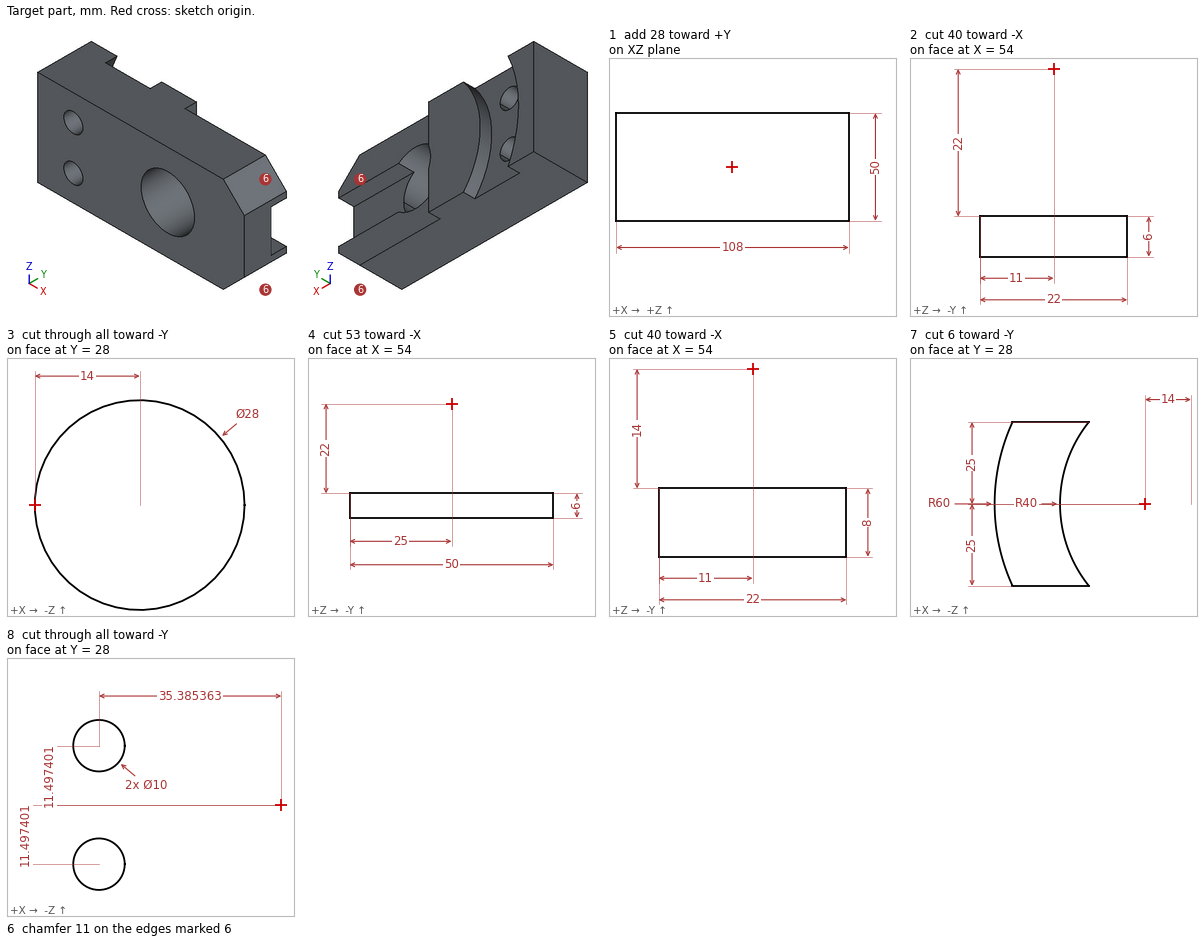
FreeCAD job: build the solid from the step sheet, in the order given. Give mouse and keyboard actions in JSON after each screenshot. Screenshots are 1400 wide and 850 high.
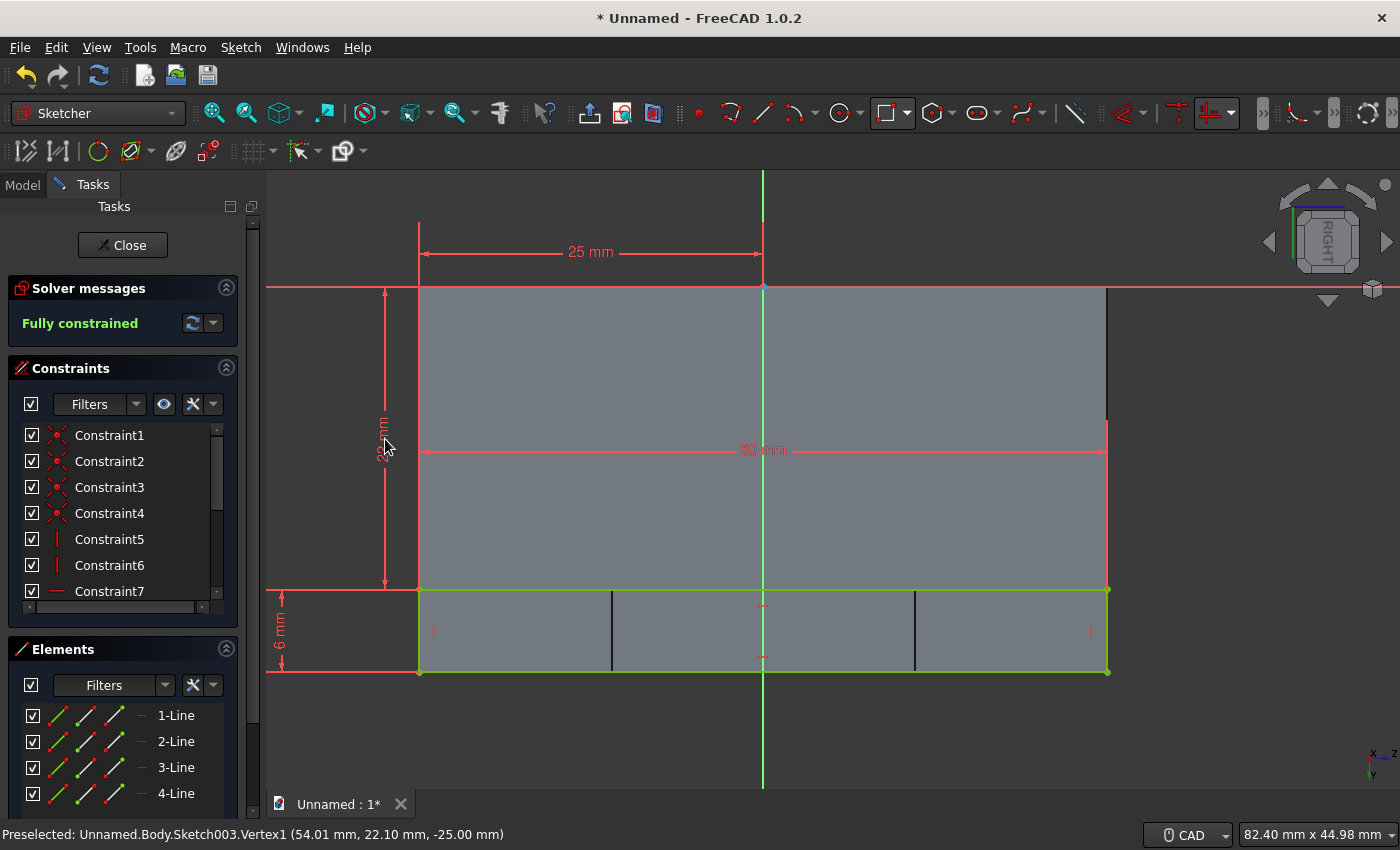
{"action": "left_click", "coordinate": [123, 245]}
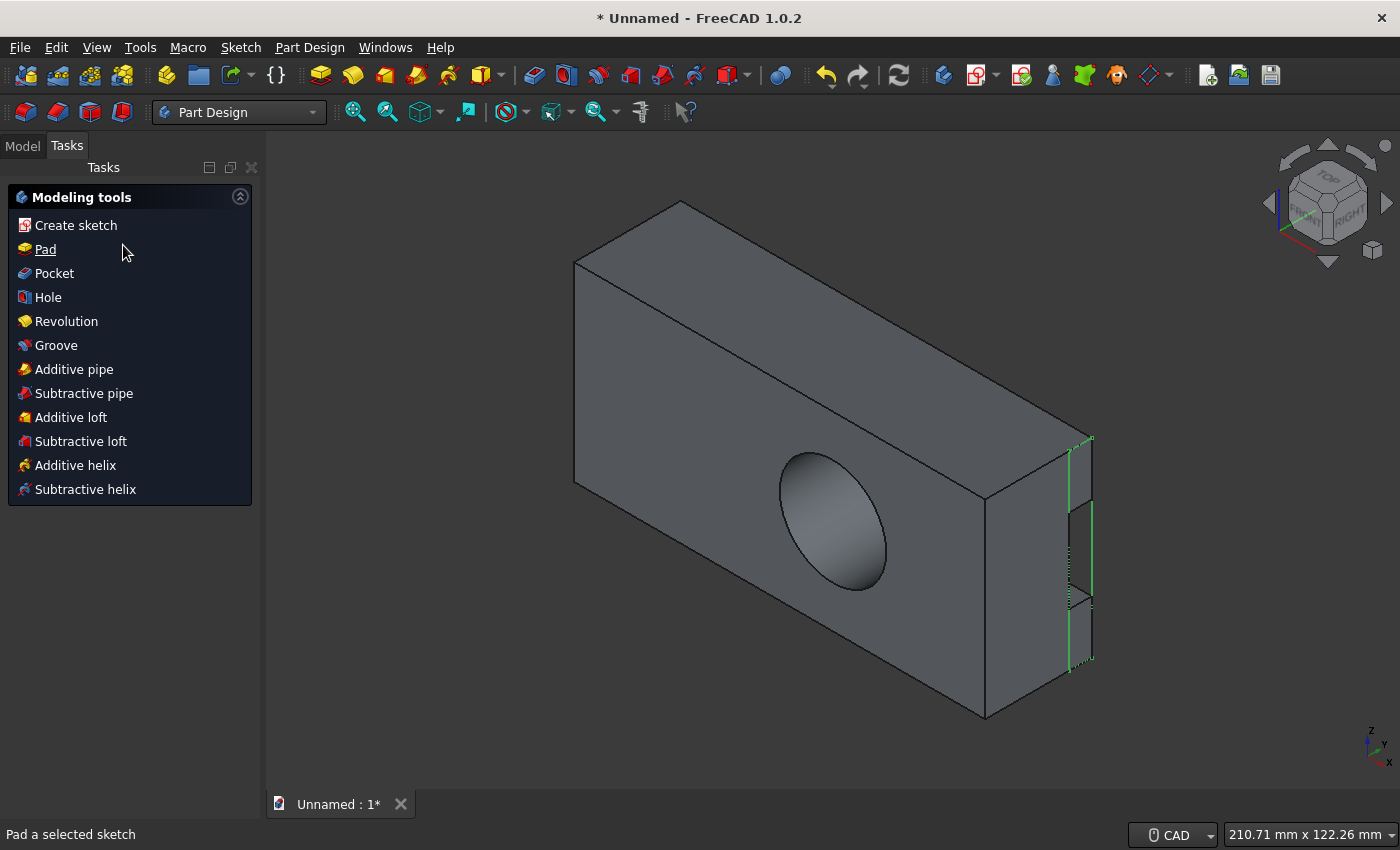
{"action": "left_click", "coordinate": [536, 76]}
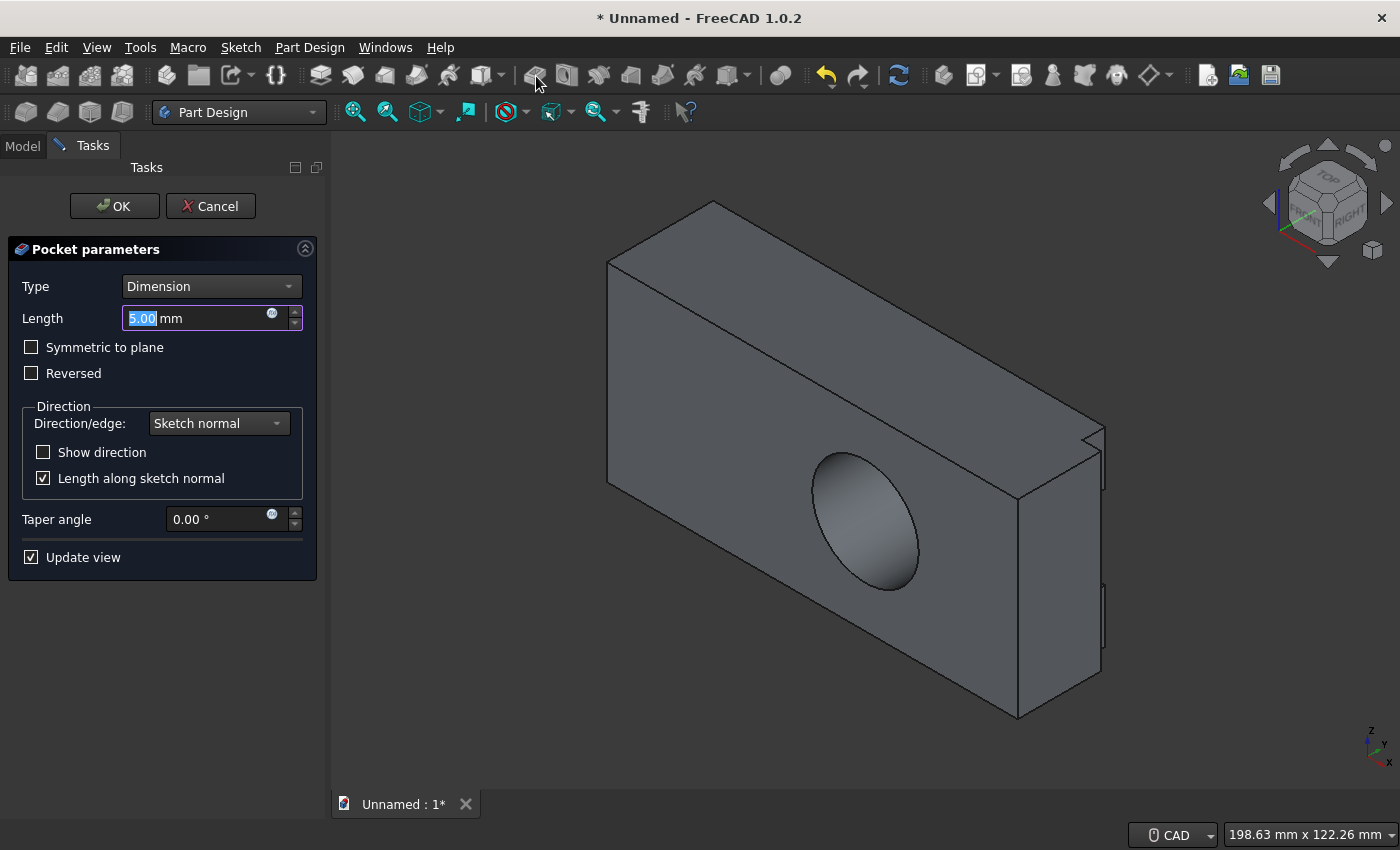
{"action": "type", "text": "53"}
{"action": "key", "text": "Tab"}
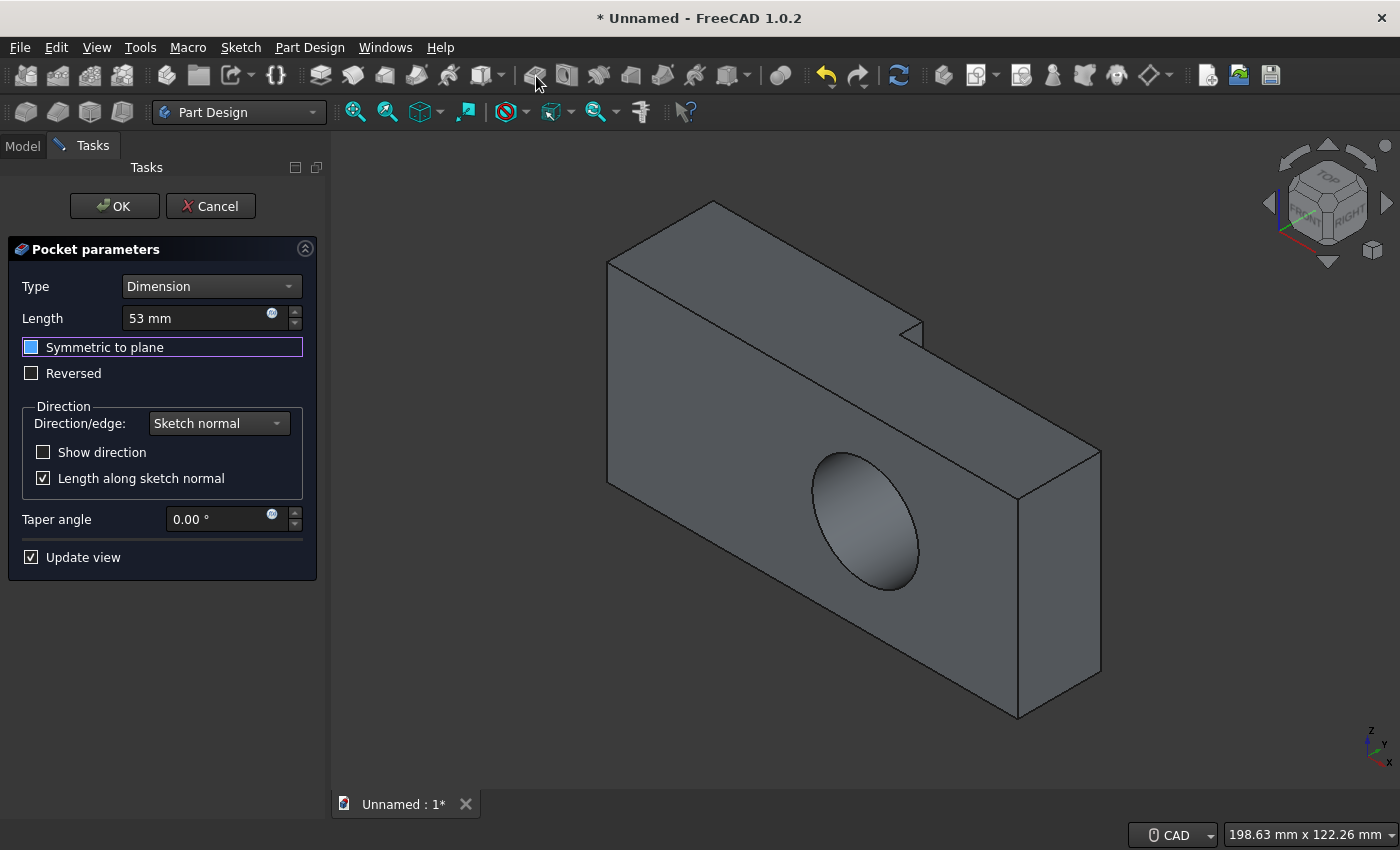
{"action": "left_click", "coordinate": [115, 206]}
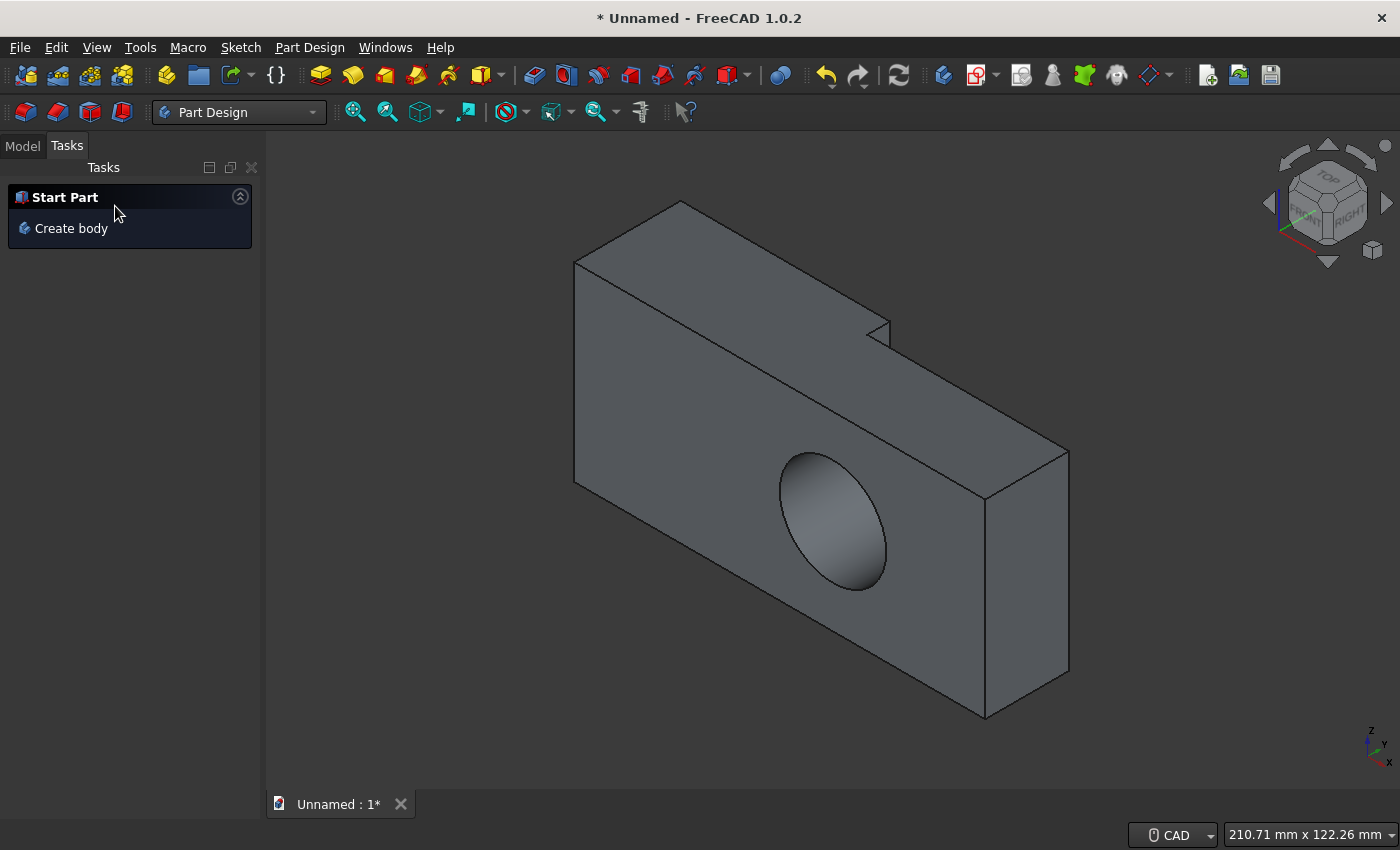
{"action": "left_click", "coordinate": [1027, 616]}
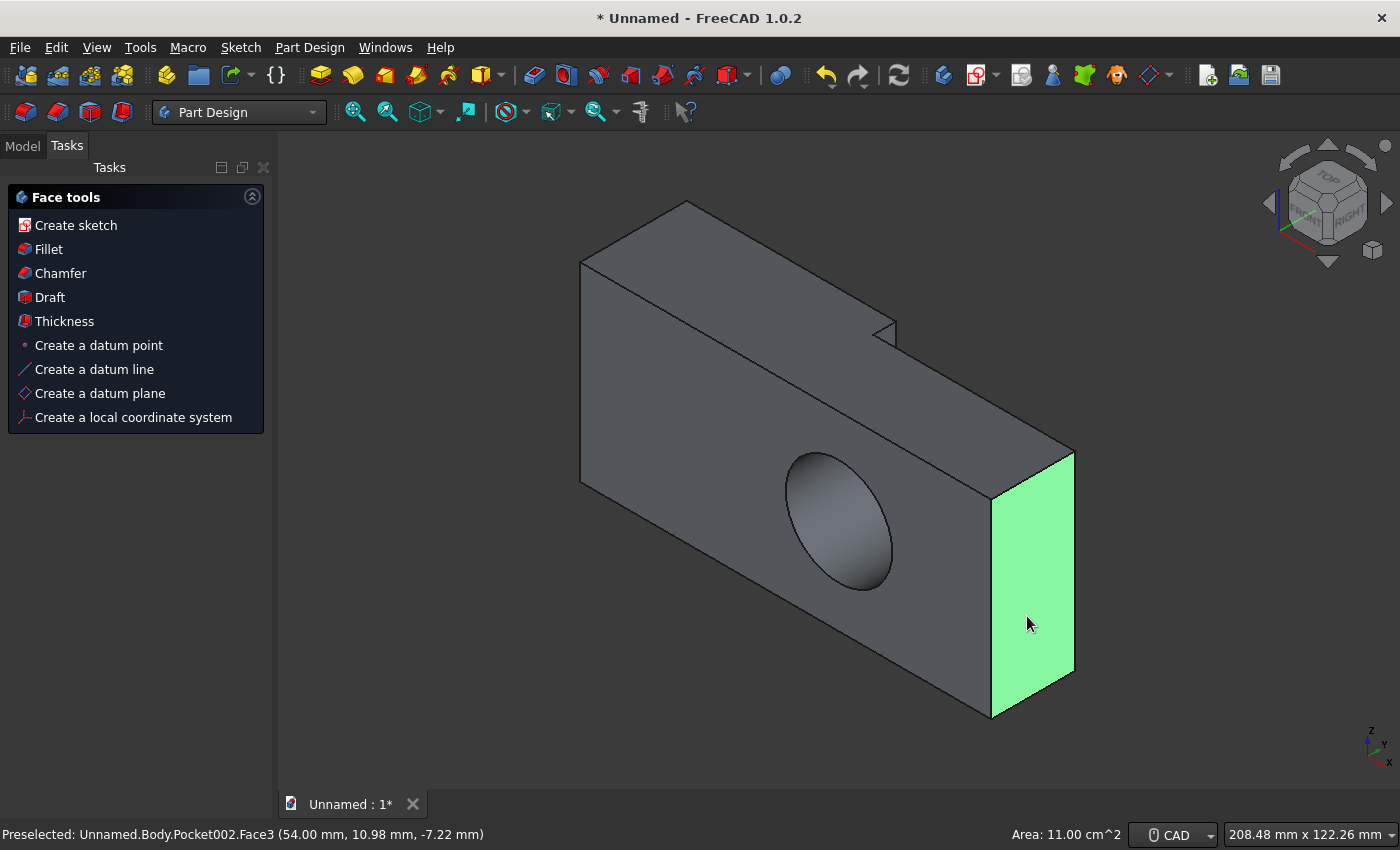
{"action": "left_click", "coordinate": [976, 76]}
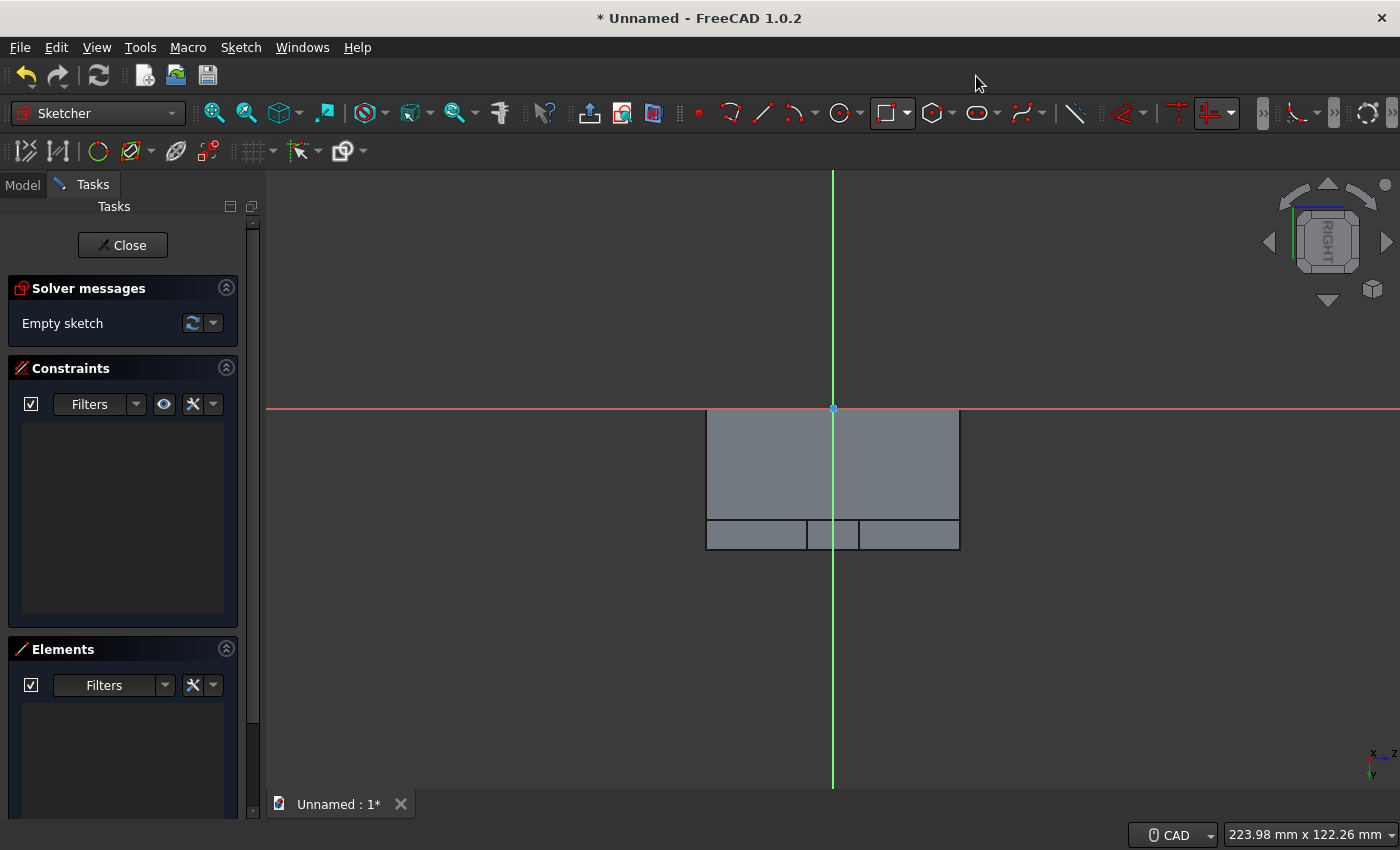
{"action": "scroll", "coordinate": [863, 458], "scroll_direction": "up", "scroll_amount": 6}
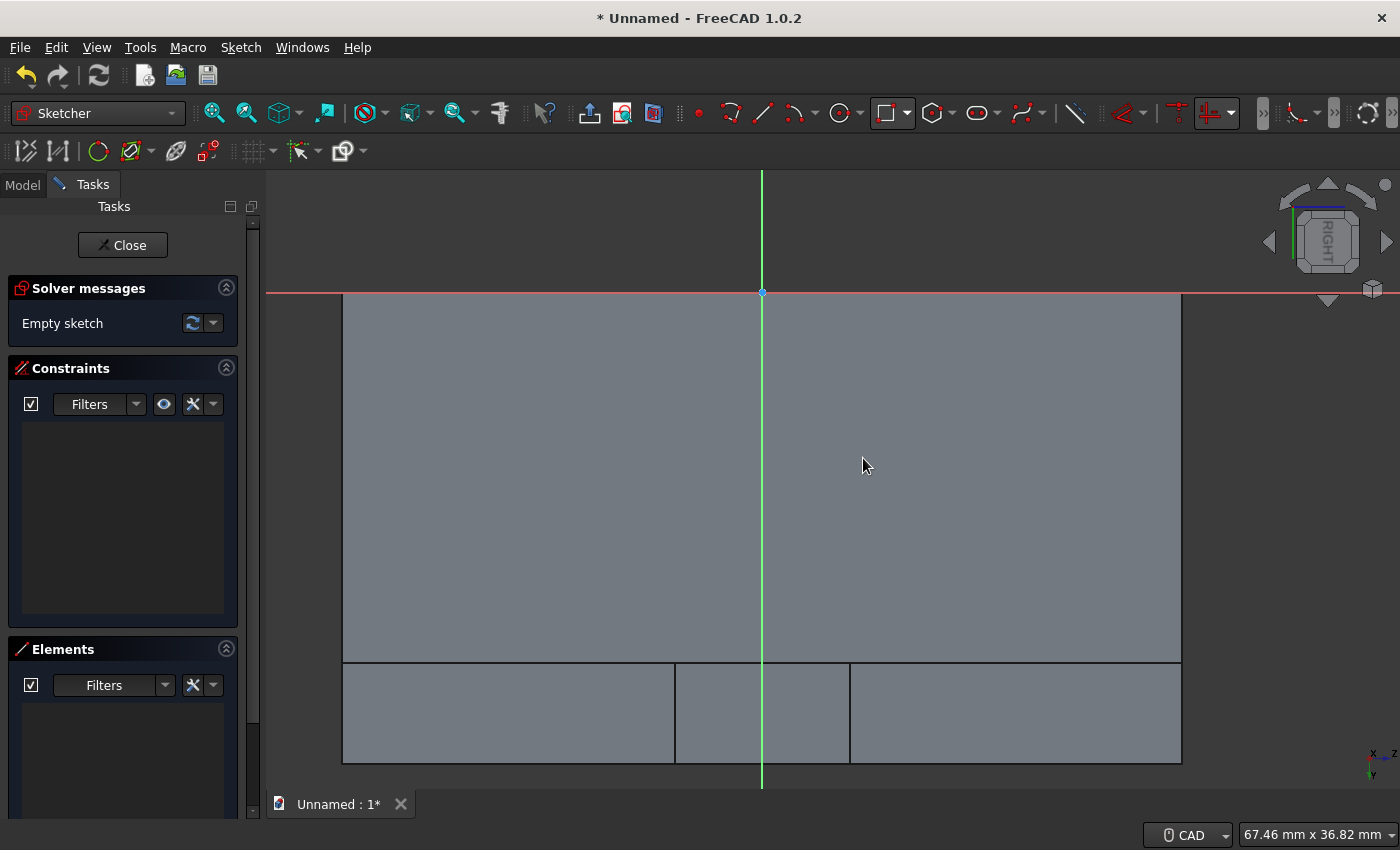
{"action": "key", "text": "g r"}